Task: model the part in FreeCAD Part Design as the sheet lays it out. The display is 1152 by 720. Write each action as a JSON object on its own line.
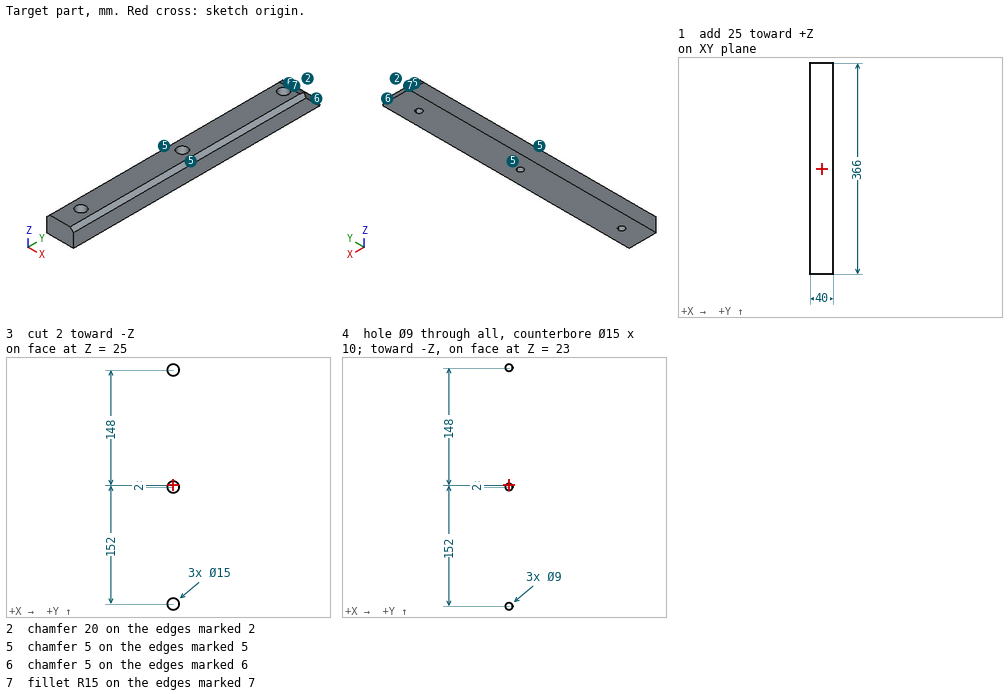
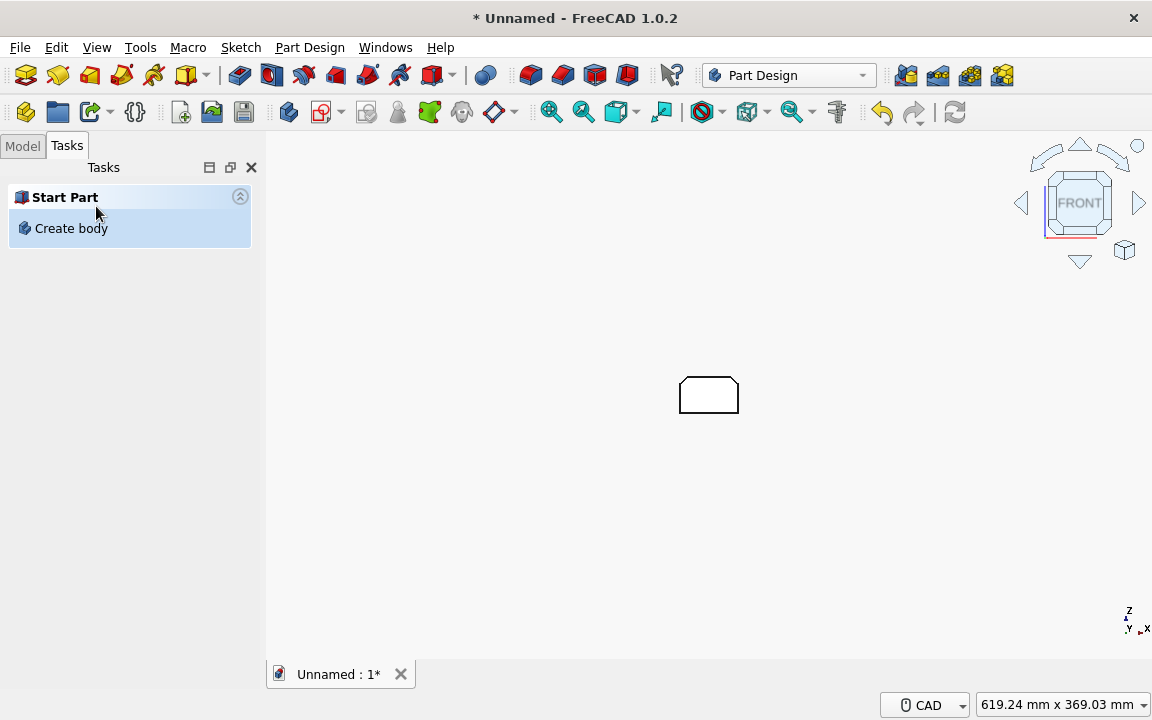
{"action": "left_click", "coordinate": [552, 112]}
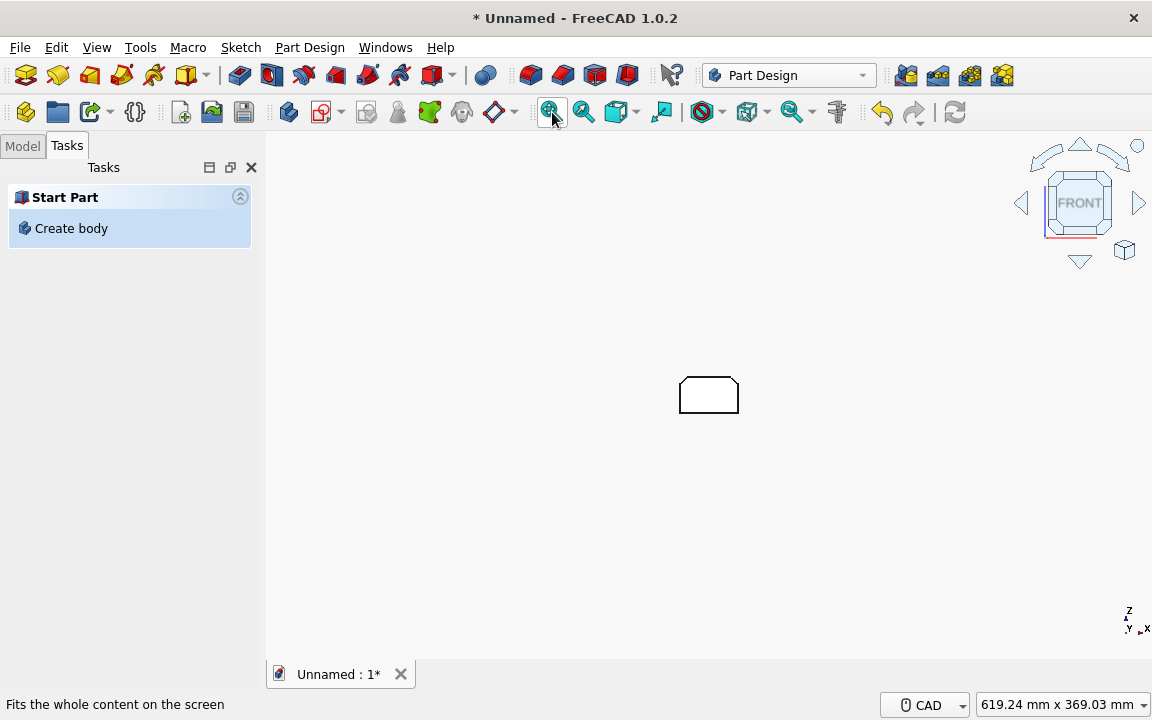
{"action": "key", "text": "3"}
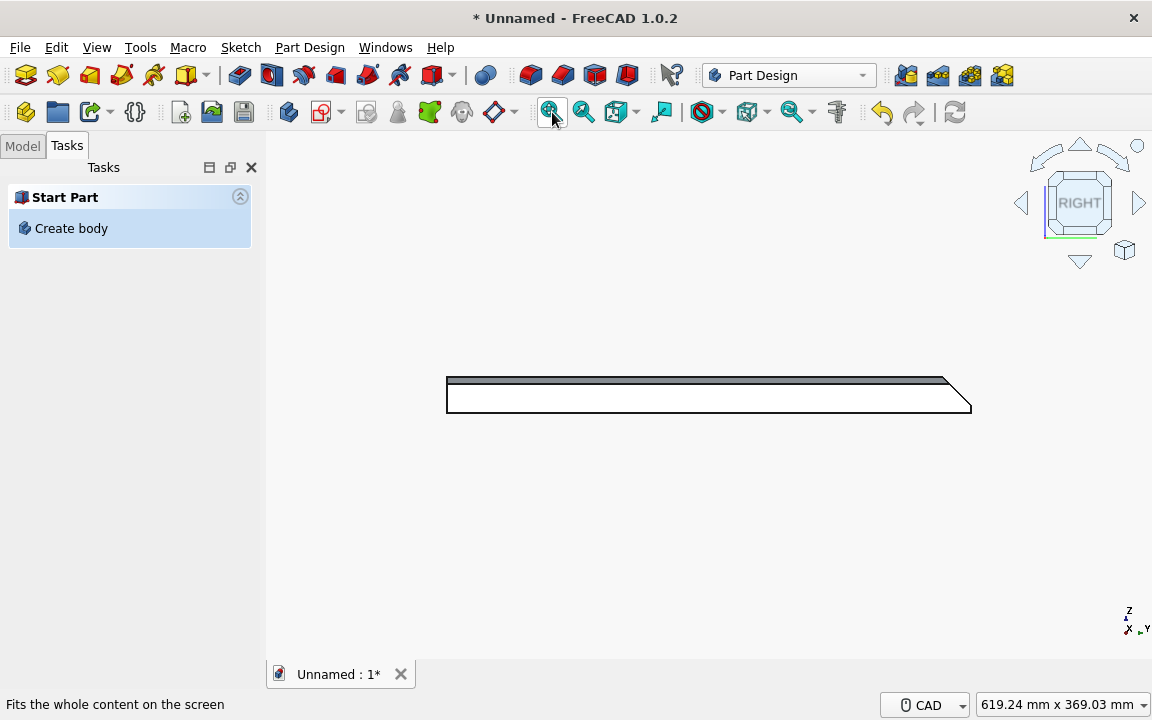
{"action": "left_click", "coordinate": [960, 394]}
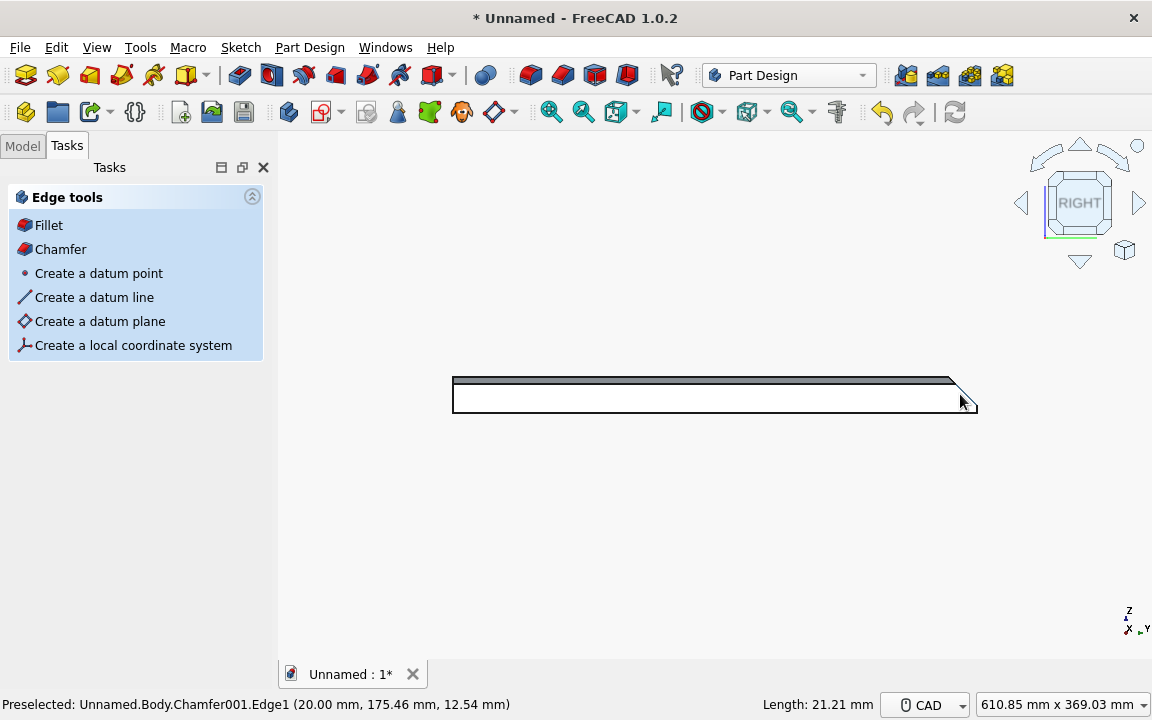
{"action": "key", "text": "5"}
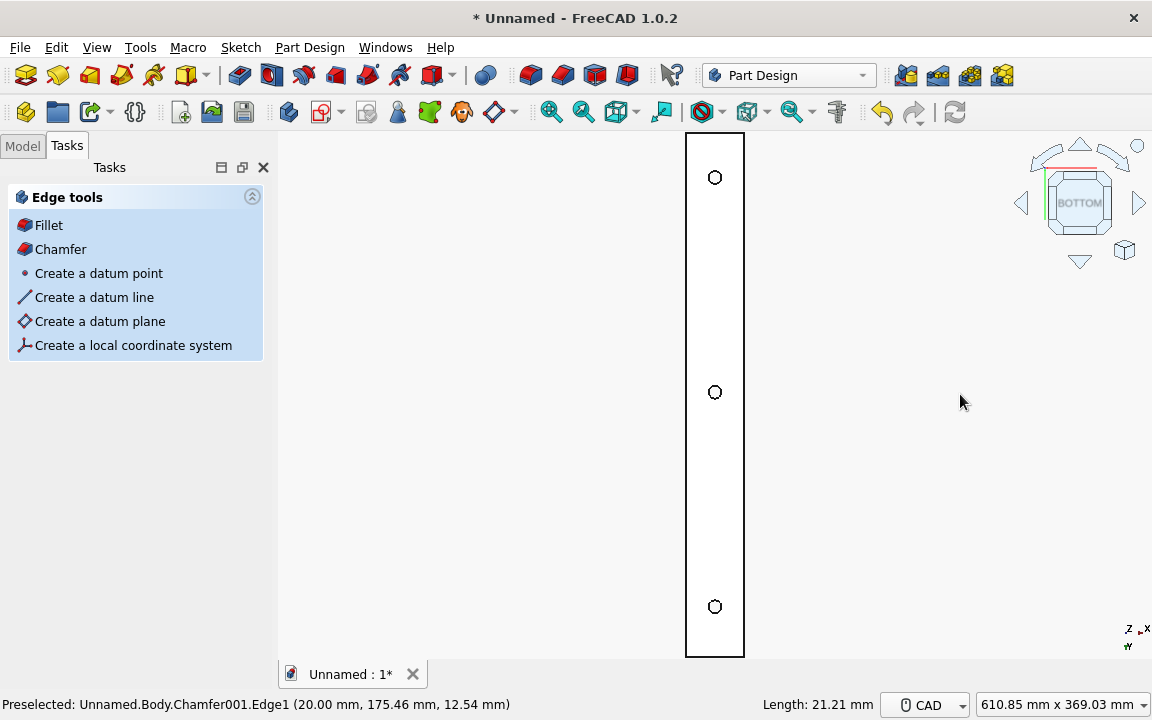
{"action": "key", "text": "4"}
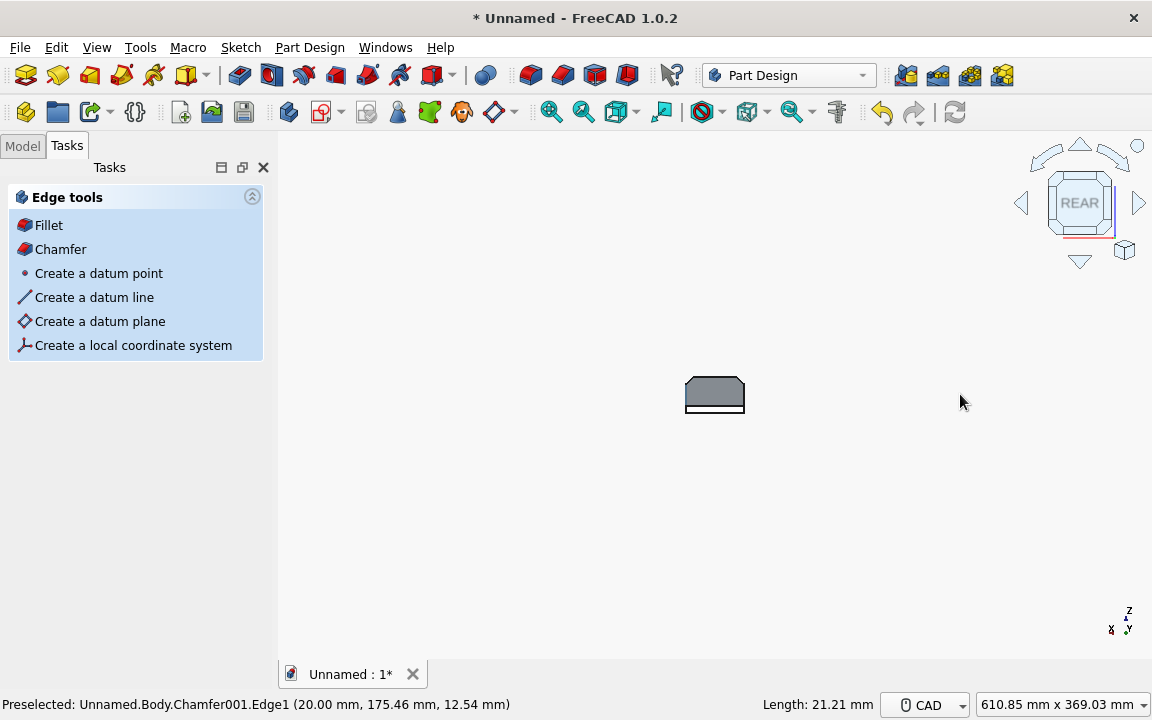
{"action": "left_click", "coordinate": [552, 112]}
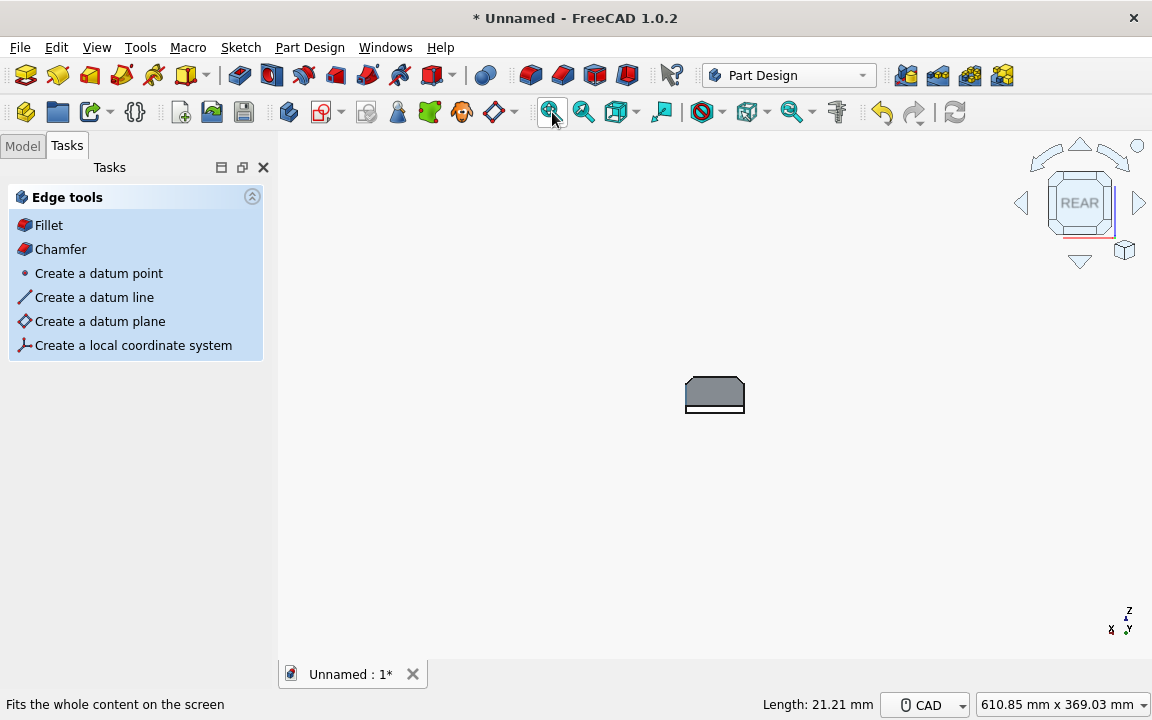
{"action": "left_click", "coordinate": [744, 394], "text": "ctrl"}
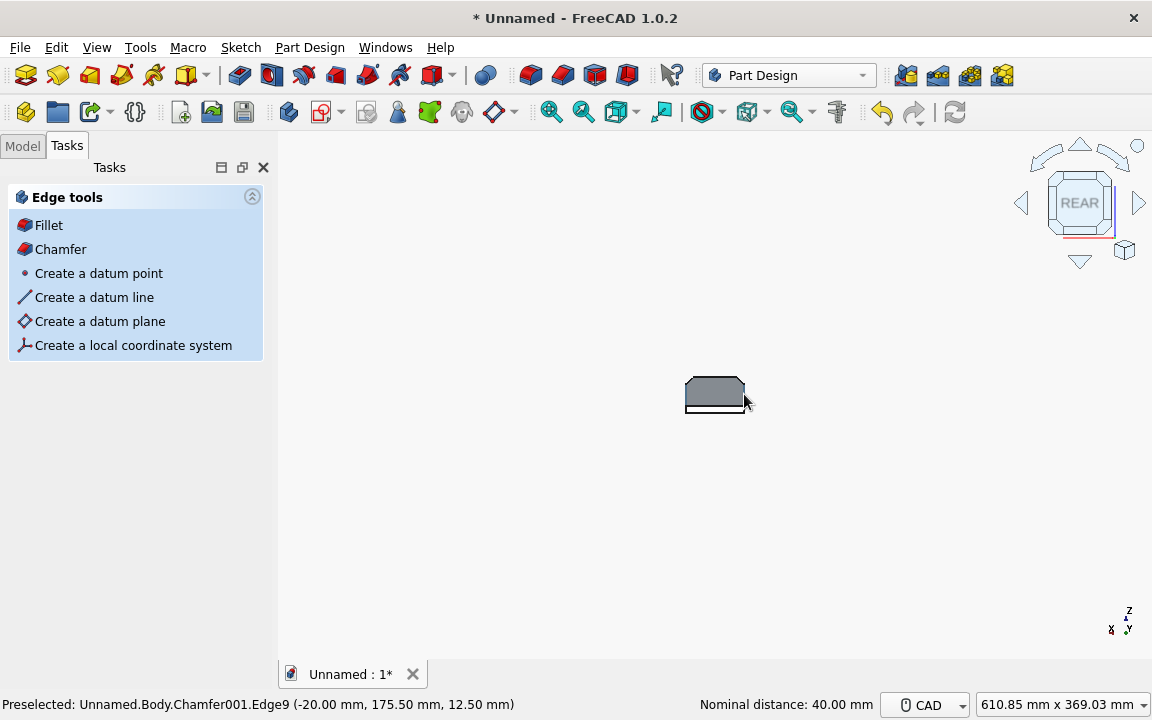
{"action": "left_click", "coordinate": [564, 76]}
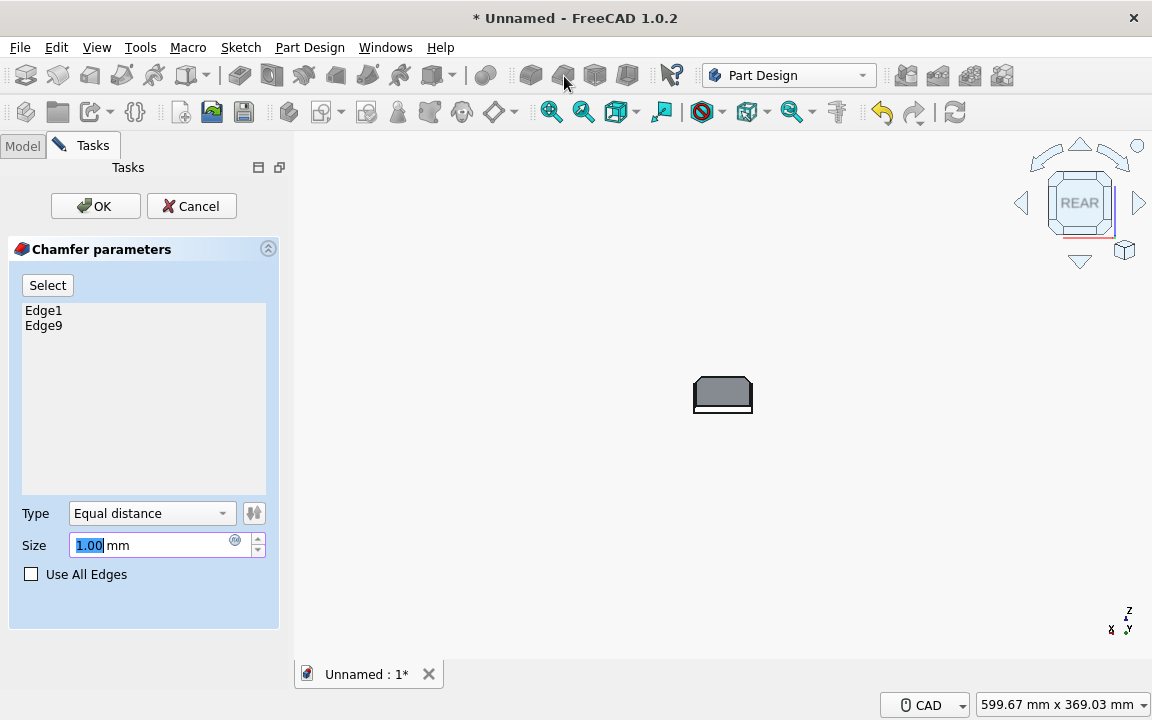
{"action": "type", "text": "5"}
{"action": "key", "text": "Tab"}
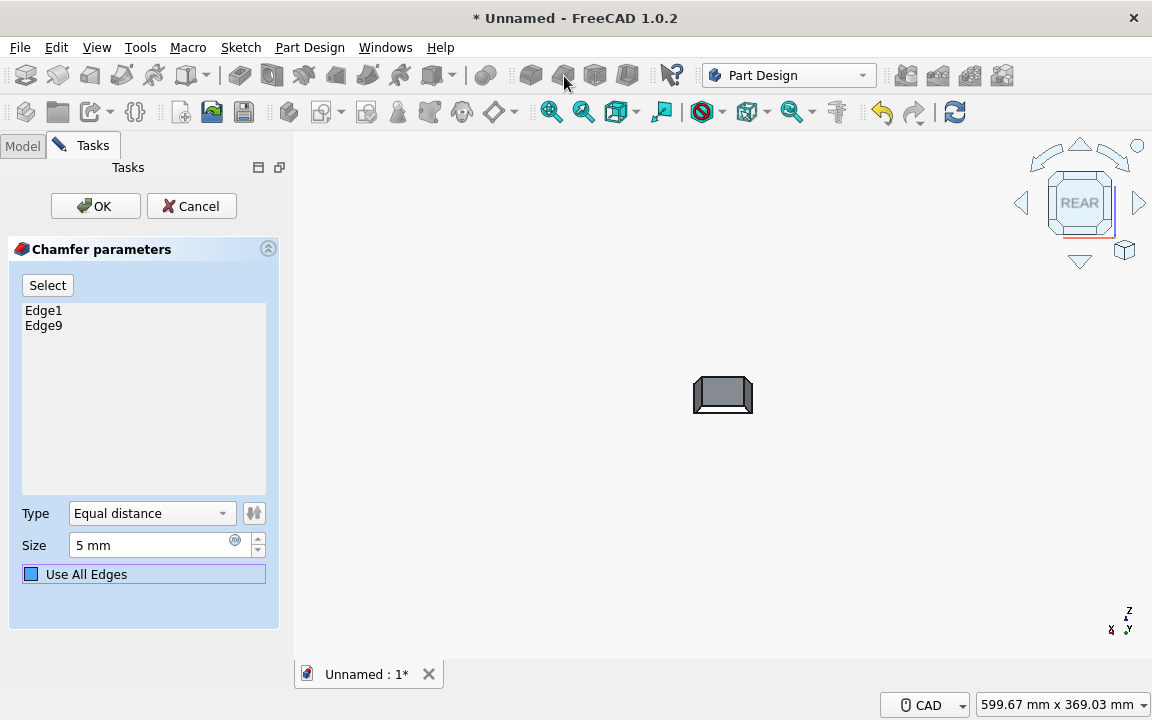
{"action": "left_click", "coordinate": [96, 206]}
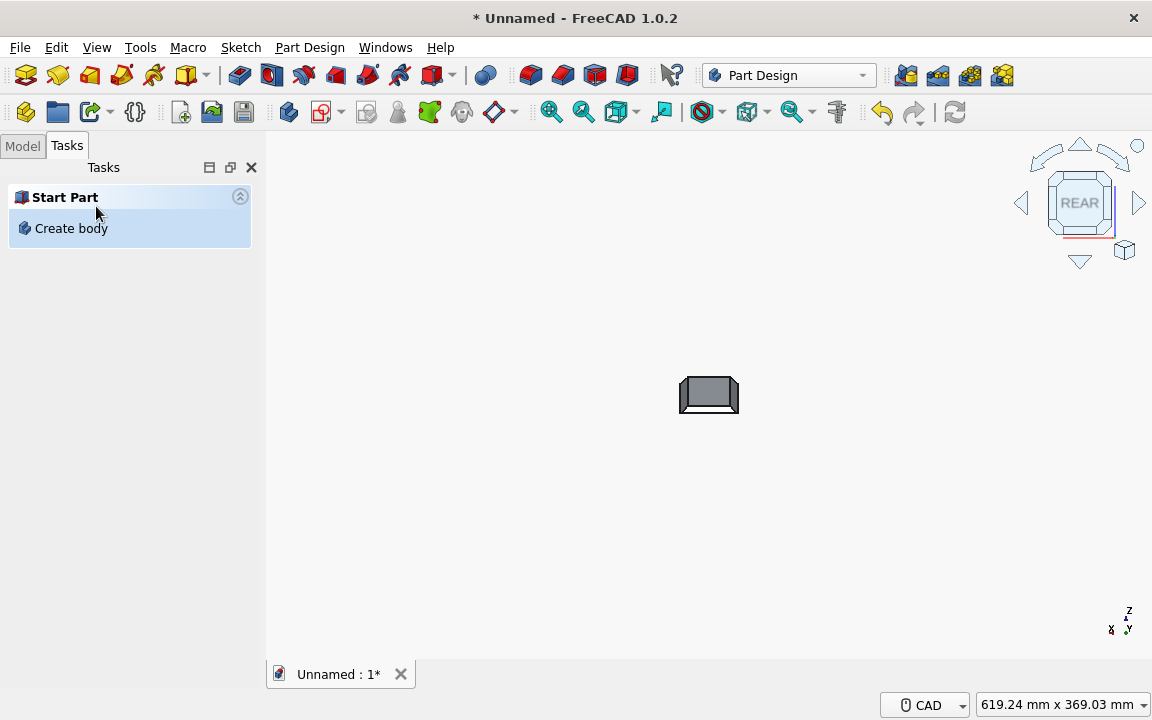
{"action": "left_click", "coordinate": [552, 112]}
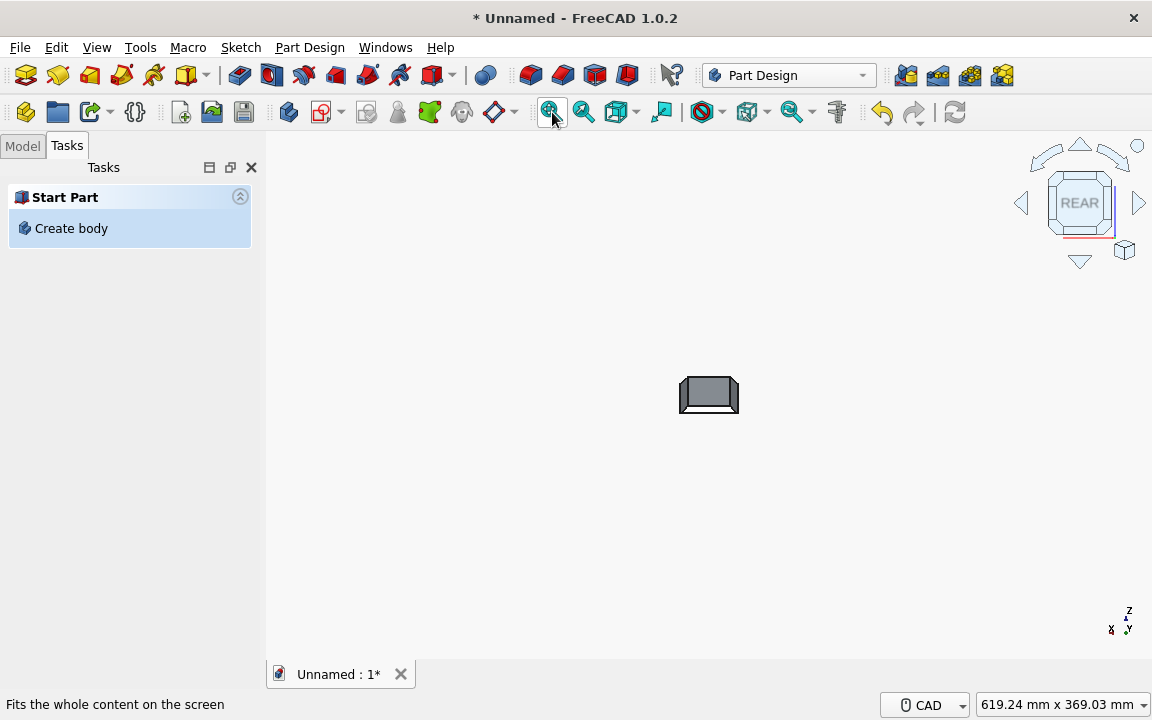
{"action": "key", "text": "0"}